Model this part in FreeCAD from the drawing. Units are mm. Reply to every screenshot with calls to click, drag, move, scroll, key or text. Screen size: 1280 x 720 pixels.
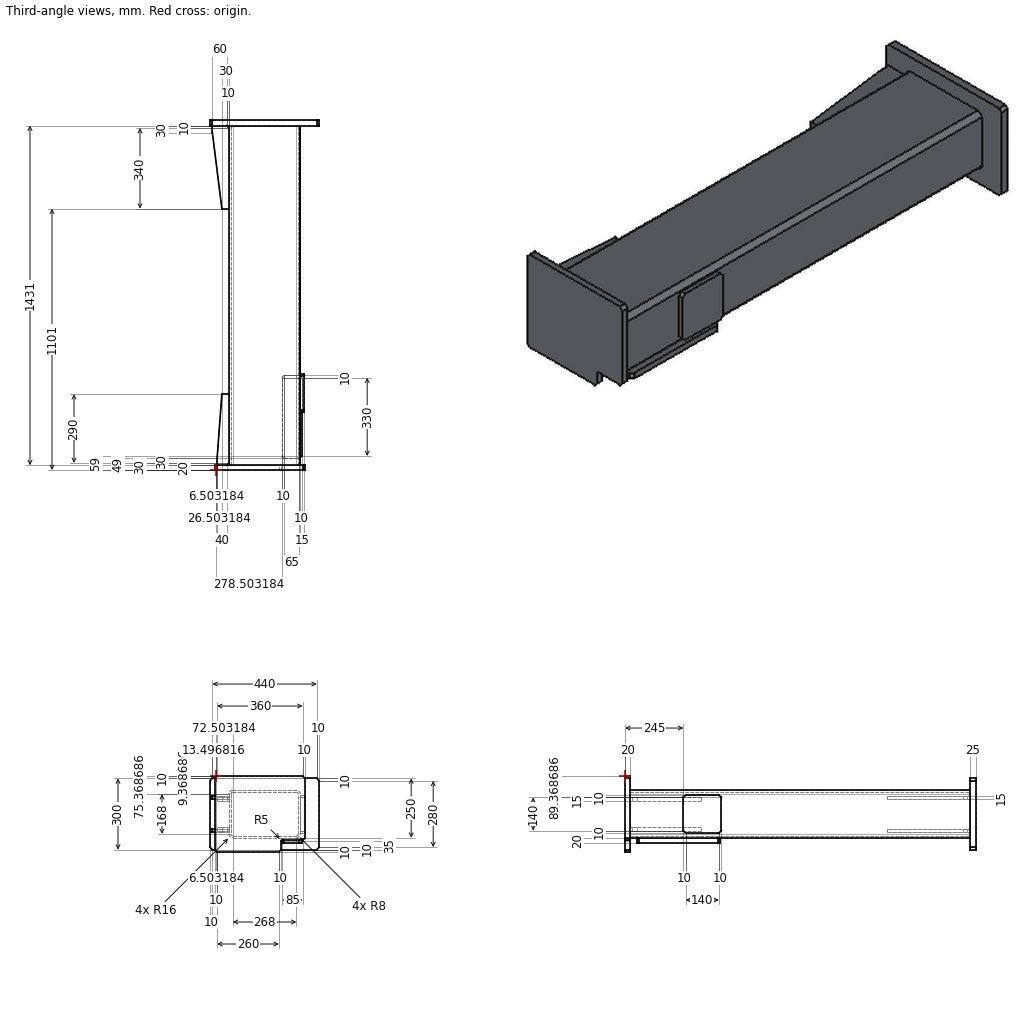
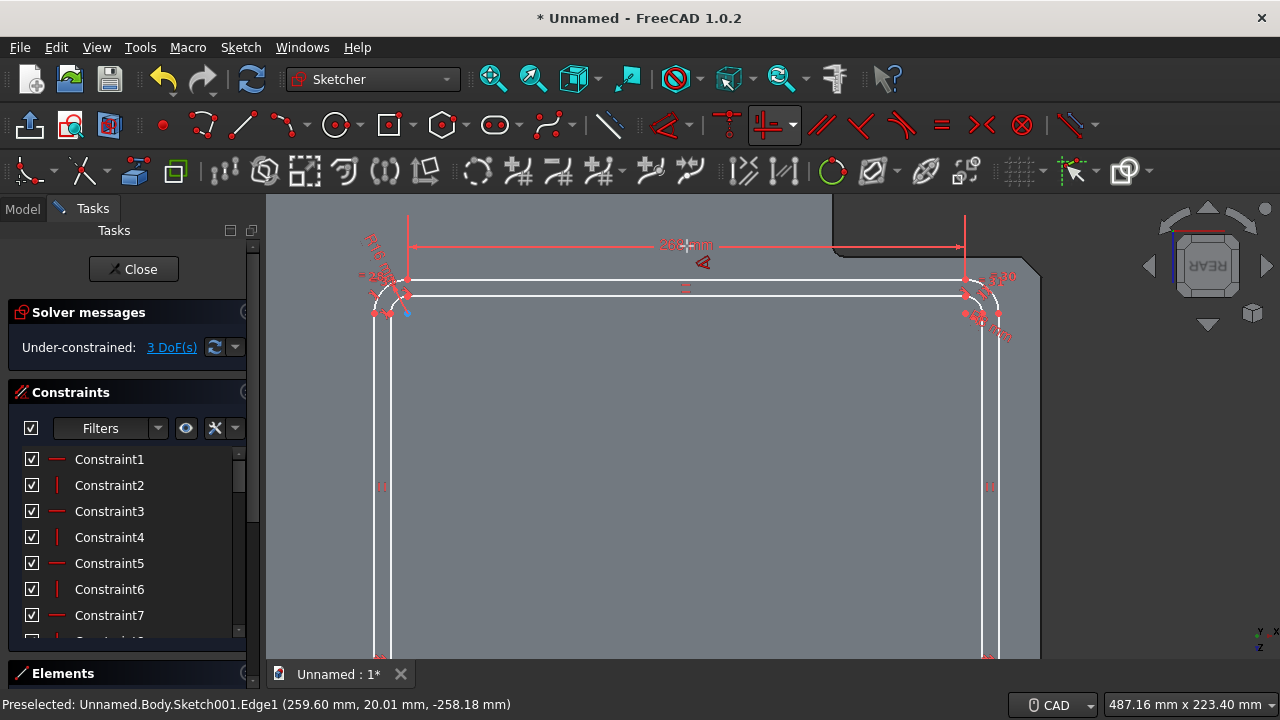
click(374, 417)
click(340, 472)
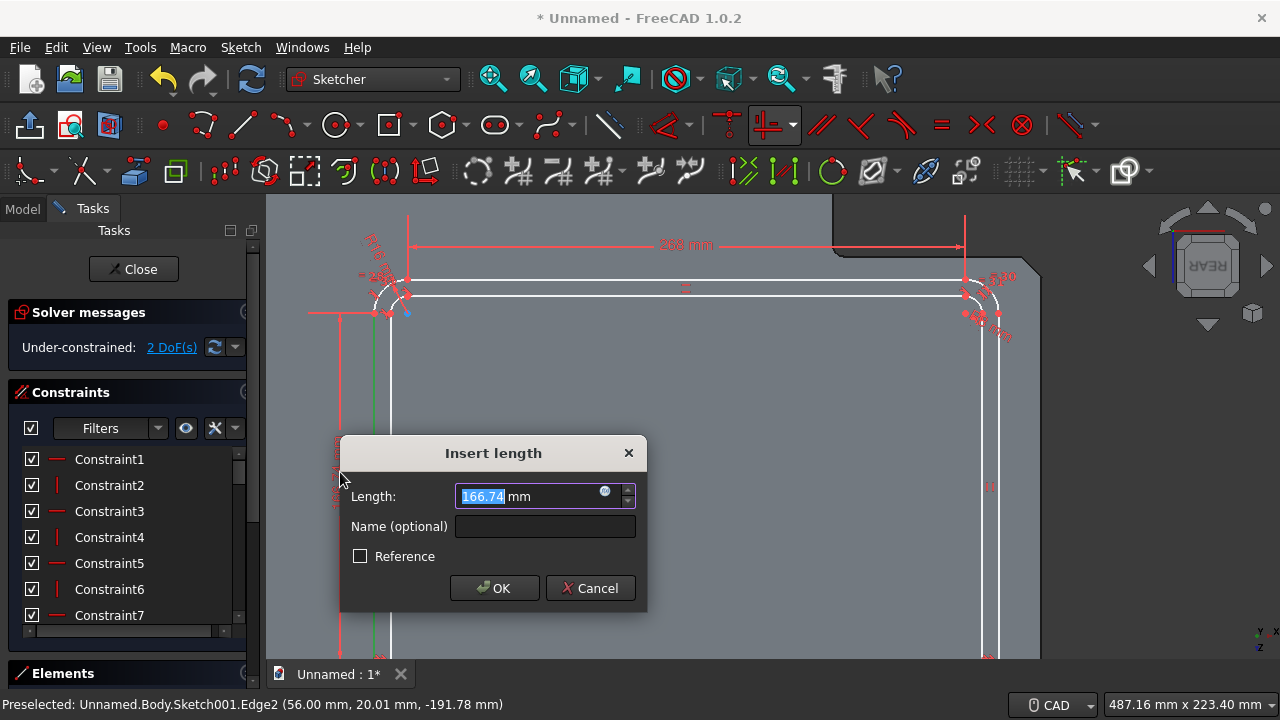
text(168)
key(Return)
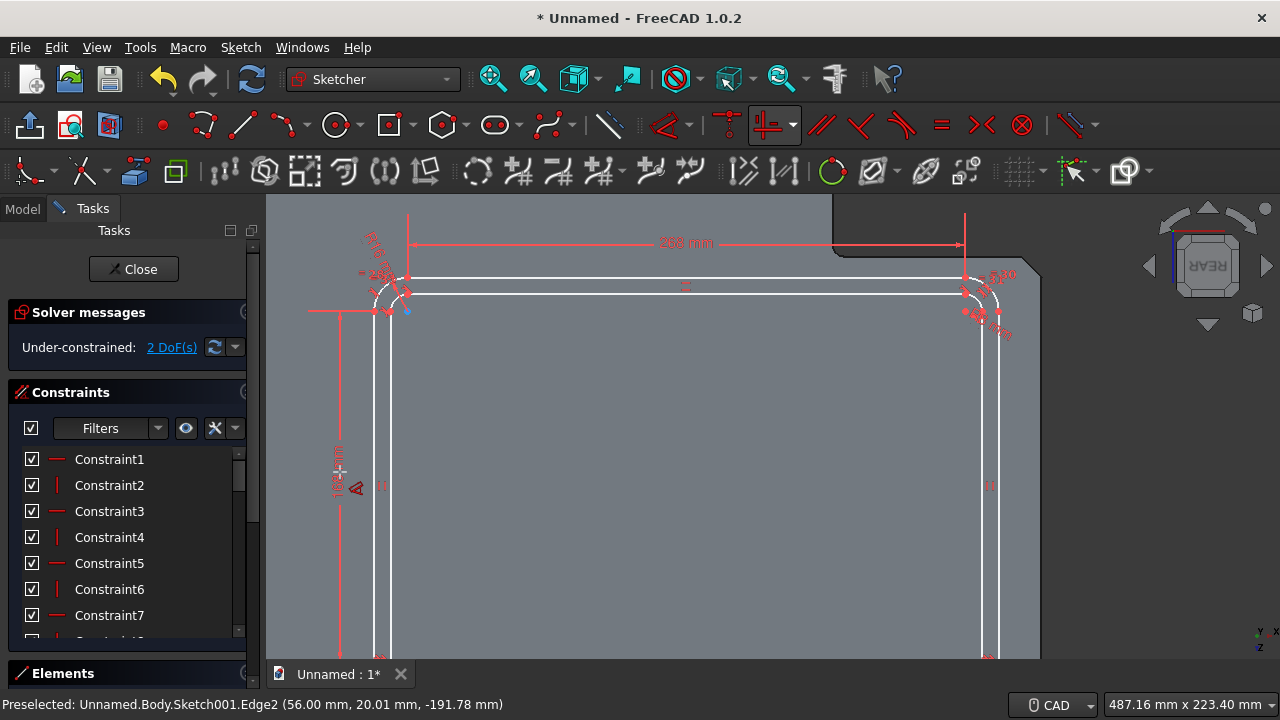
click(408, 278)
click(351, 244)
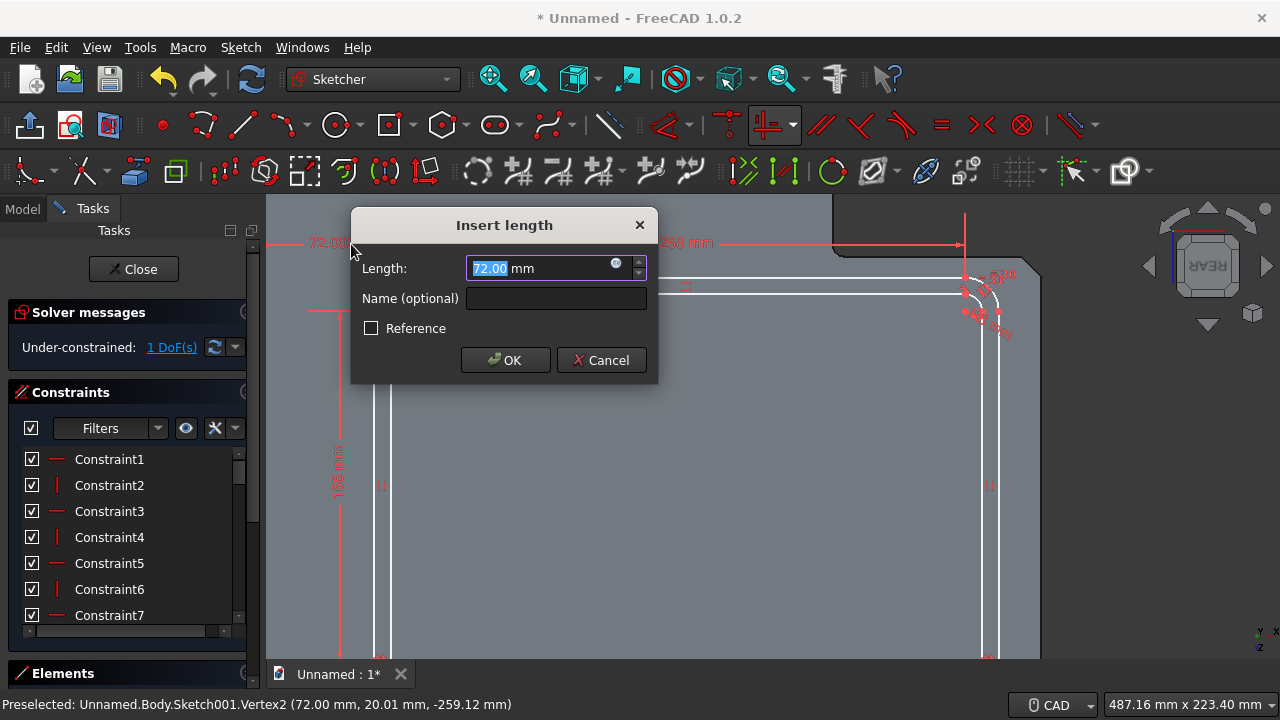
text(72.503184)
key(Return)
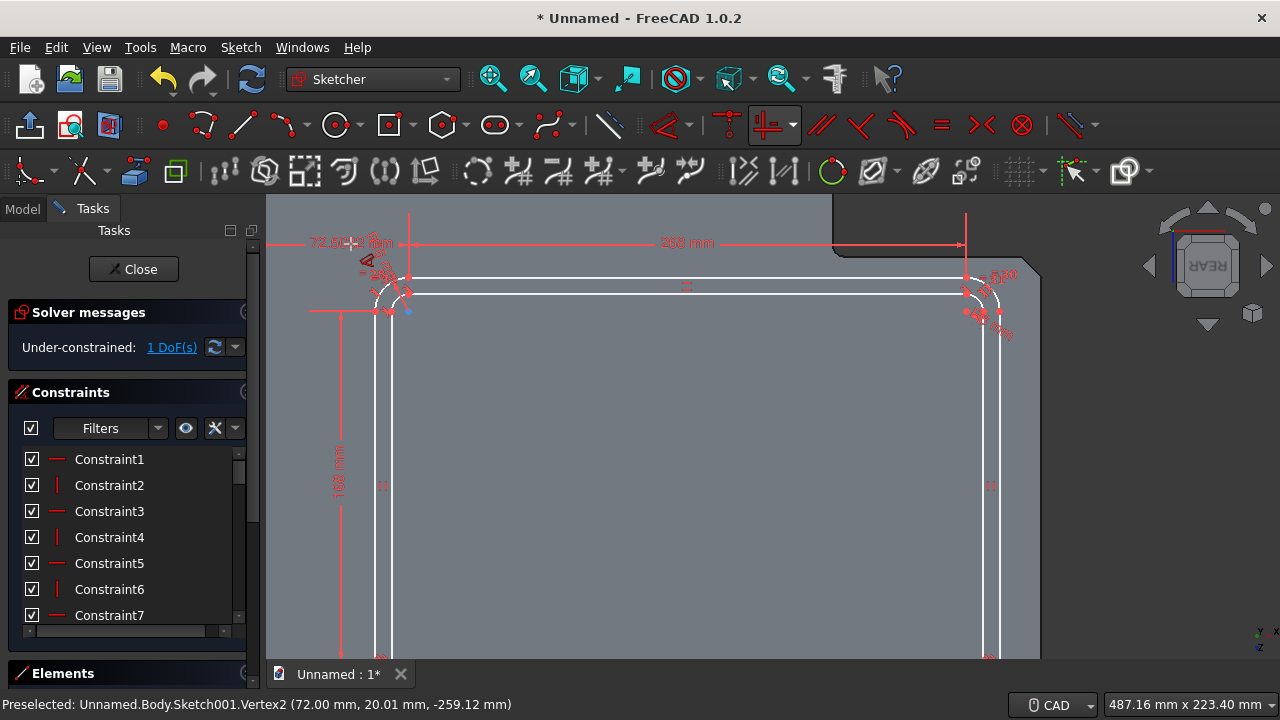
scroll(797, 280, down, 3)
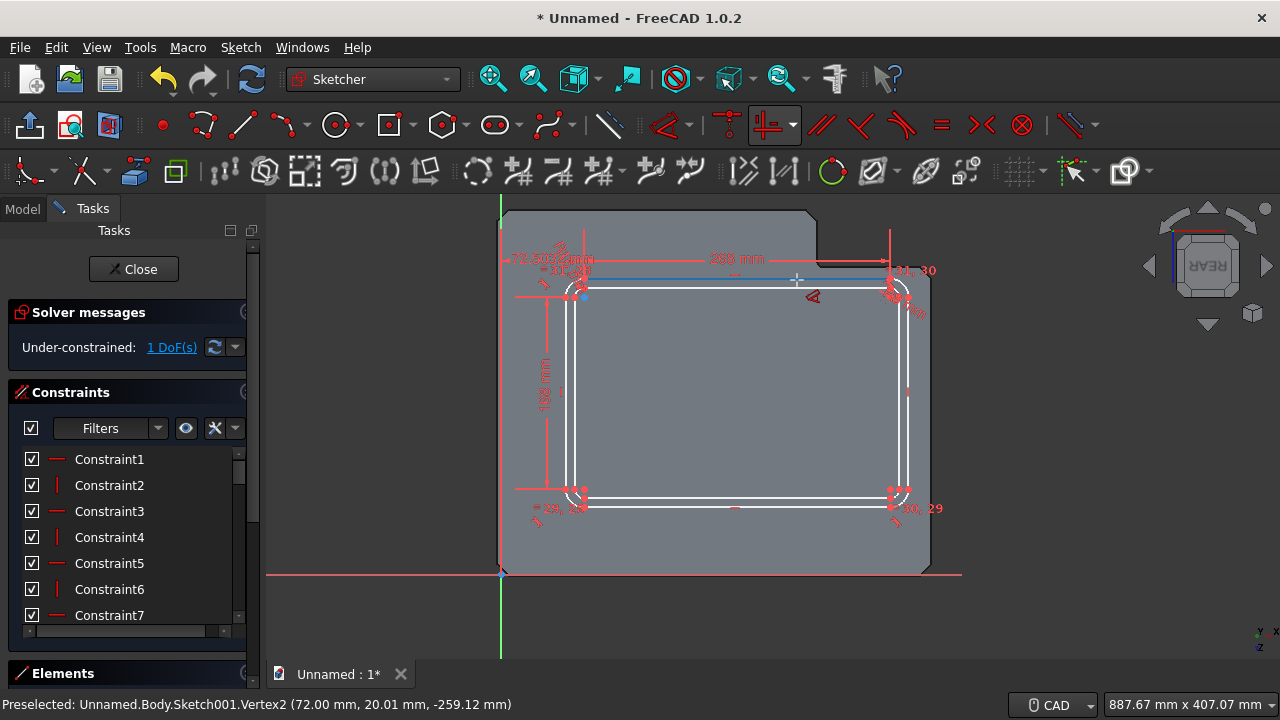
scroll(566, 489, up, 2)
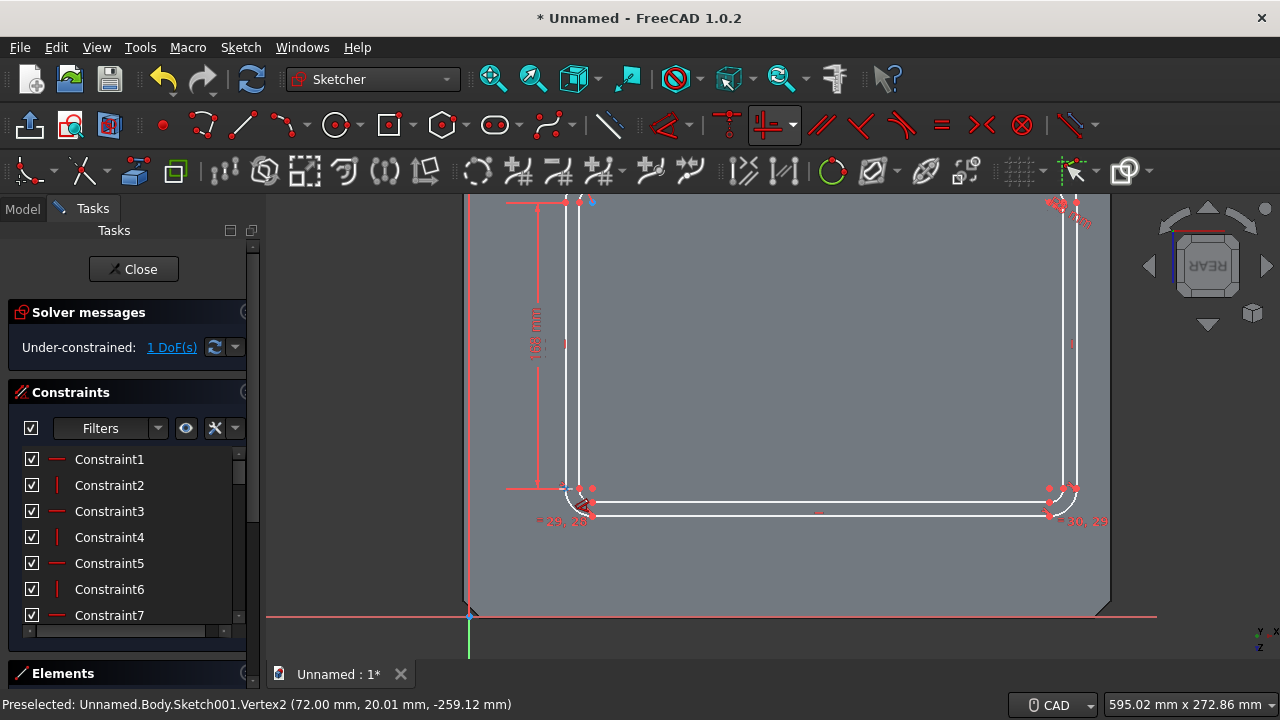
click(566, 489)
click(435, 553)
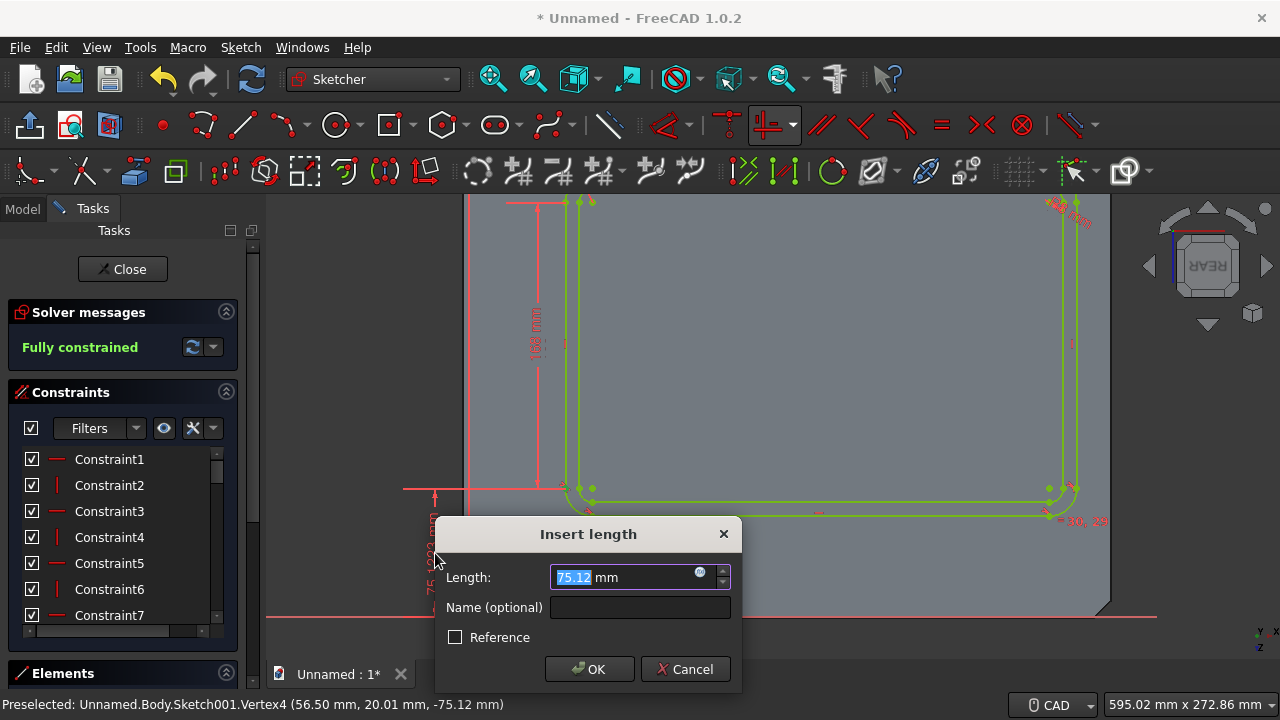
text(75.368686)
key(Return)
key(Escape)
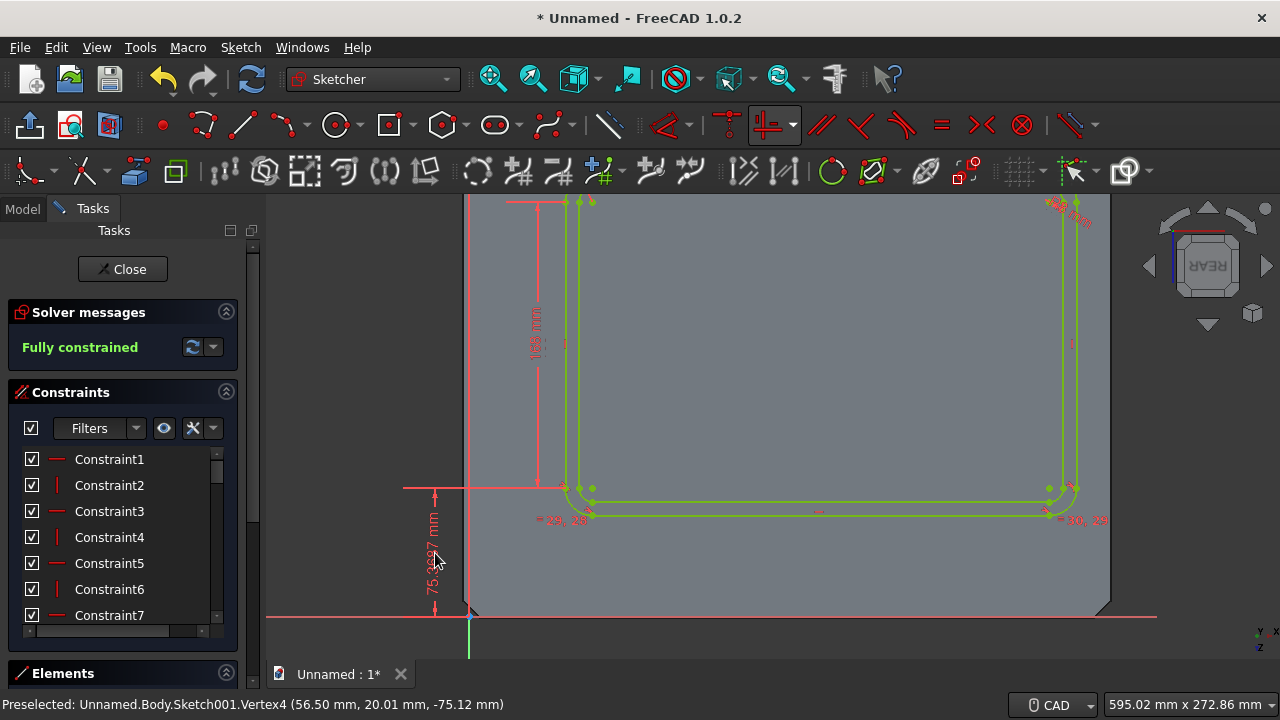
click(123, 269)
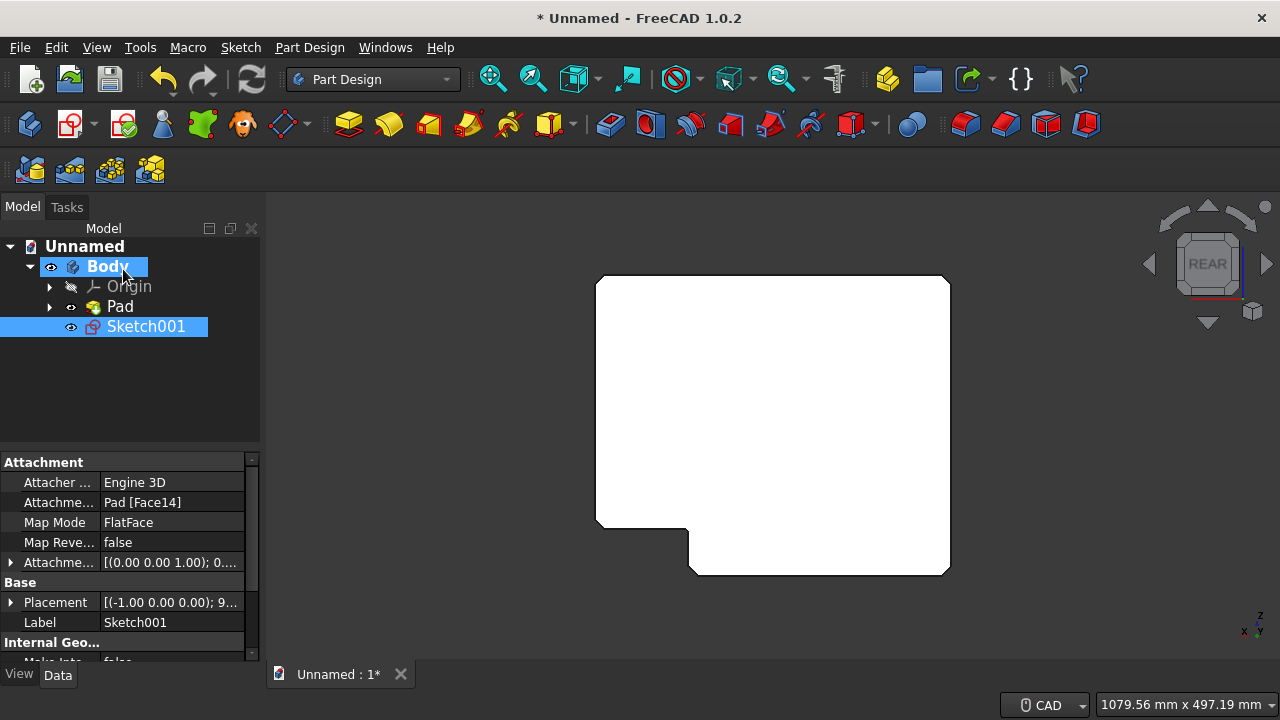
click(350, 124)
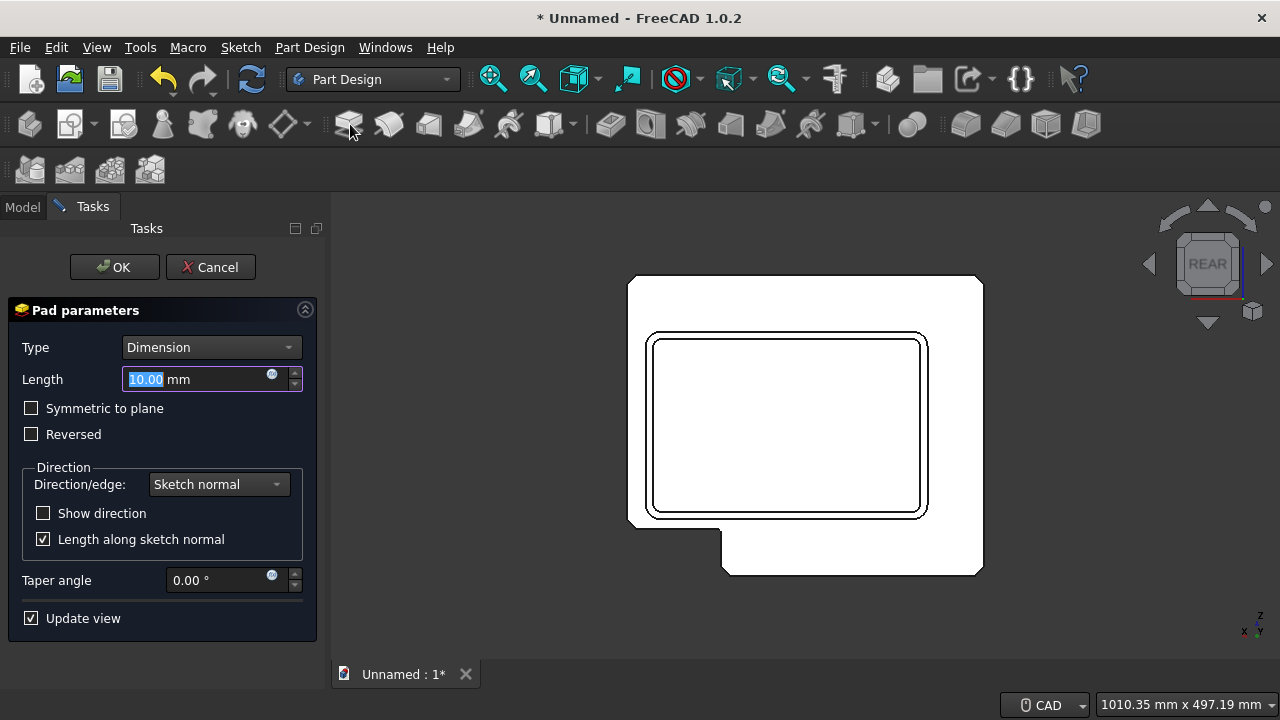
text(1431)
key(Tab)